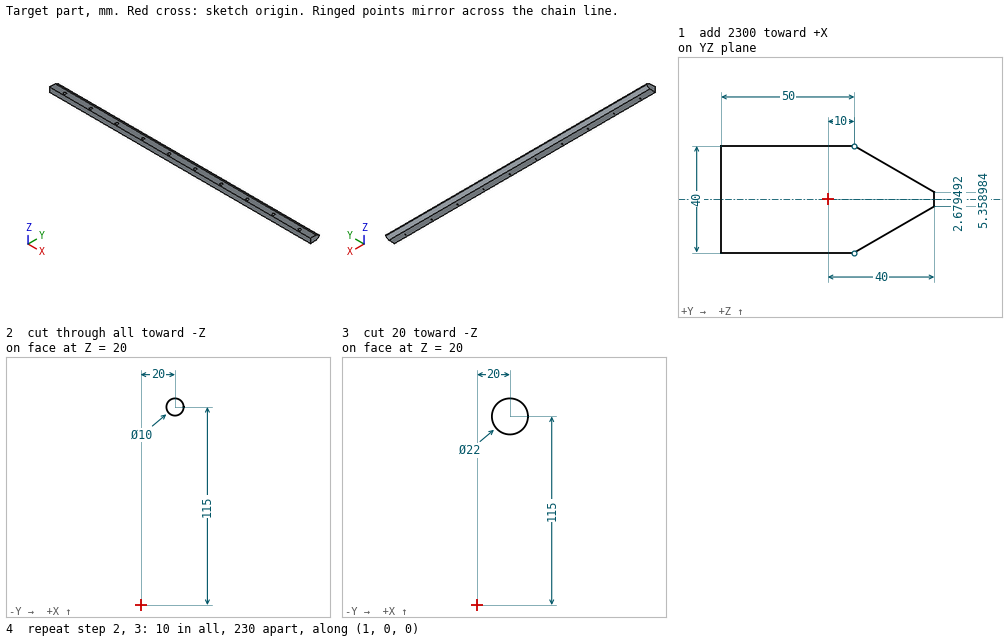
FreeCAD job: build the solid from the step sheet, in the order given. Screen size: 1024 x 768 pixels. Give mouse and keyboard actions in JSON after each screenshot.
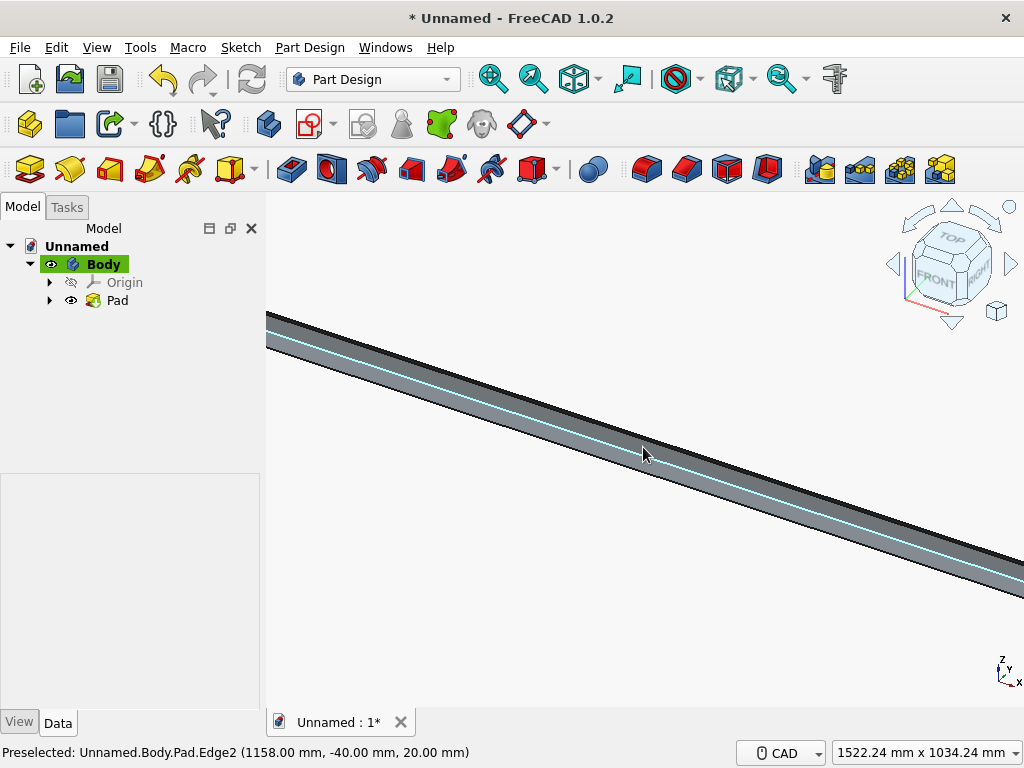
{"action": "key", "text": "v f"}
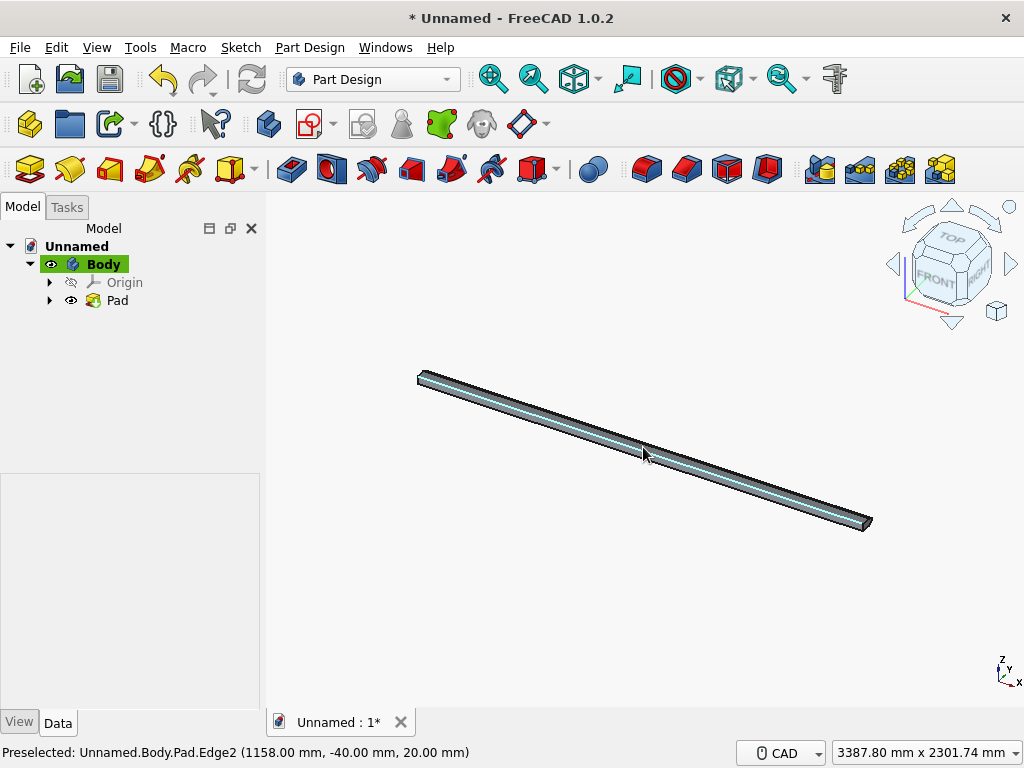
{"action": "key", "text": "0"}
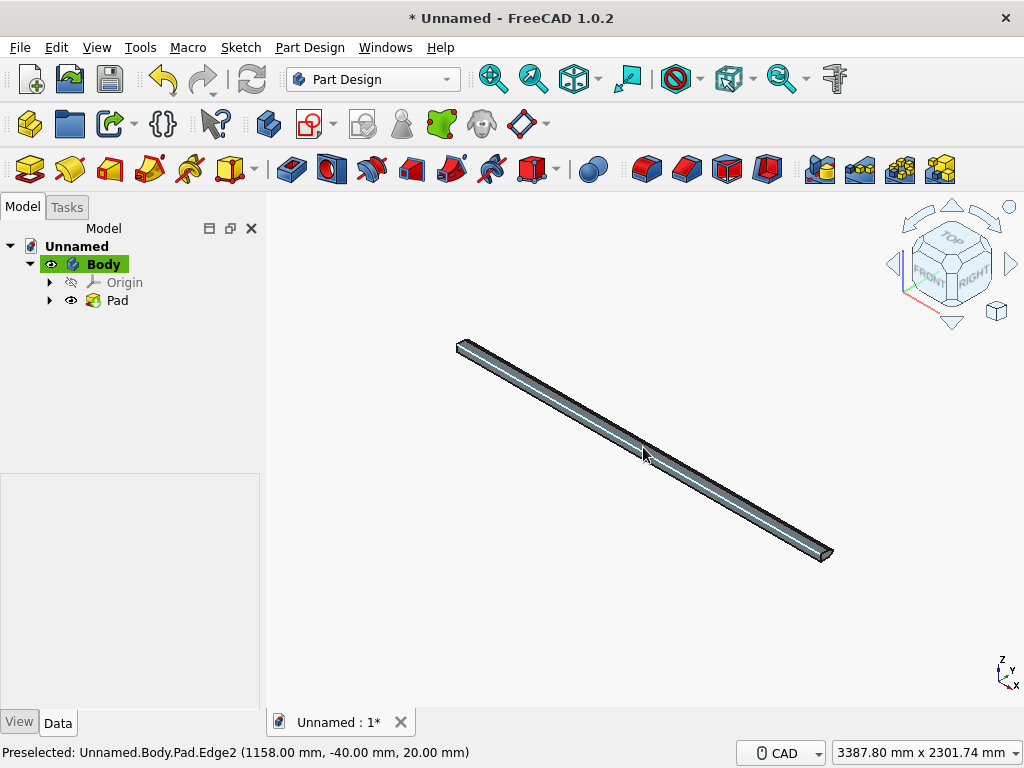
{"action": "scroll", "coordinate": [643, 446], "scroll_direction": "up", "scroll_amount": 4}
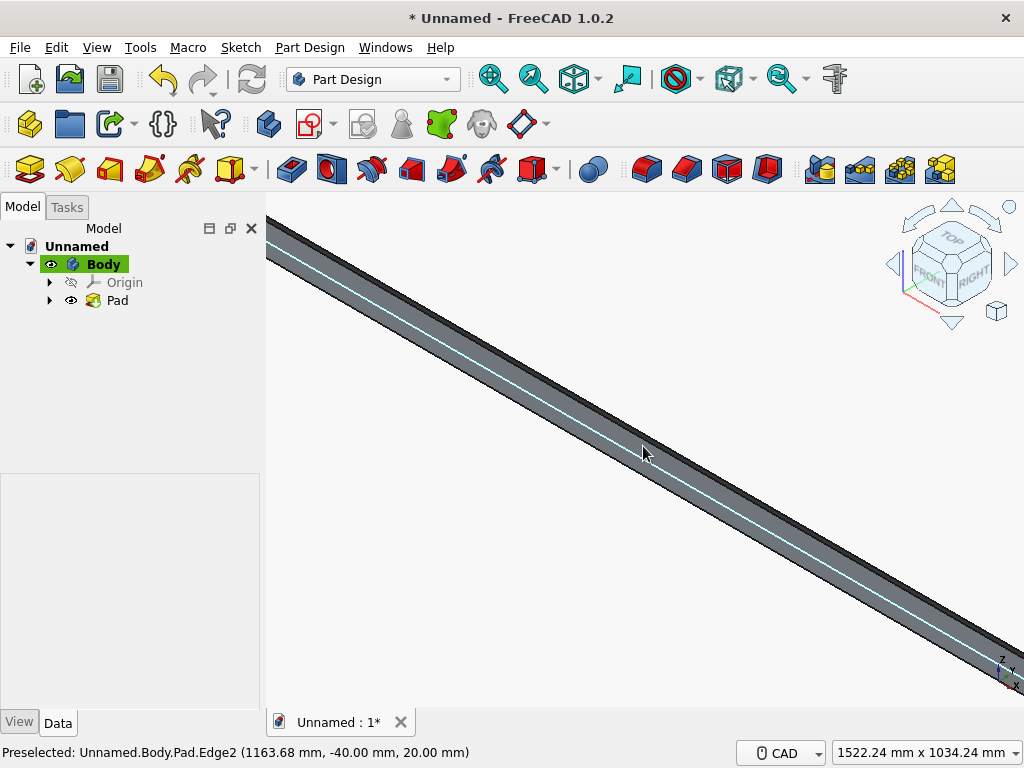
{"action": "left_click", "coordinate": [642, 447]}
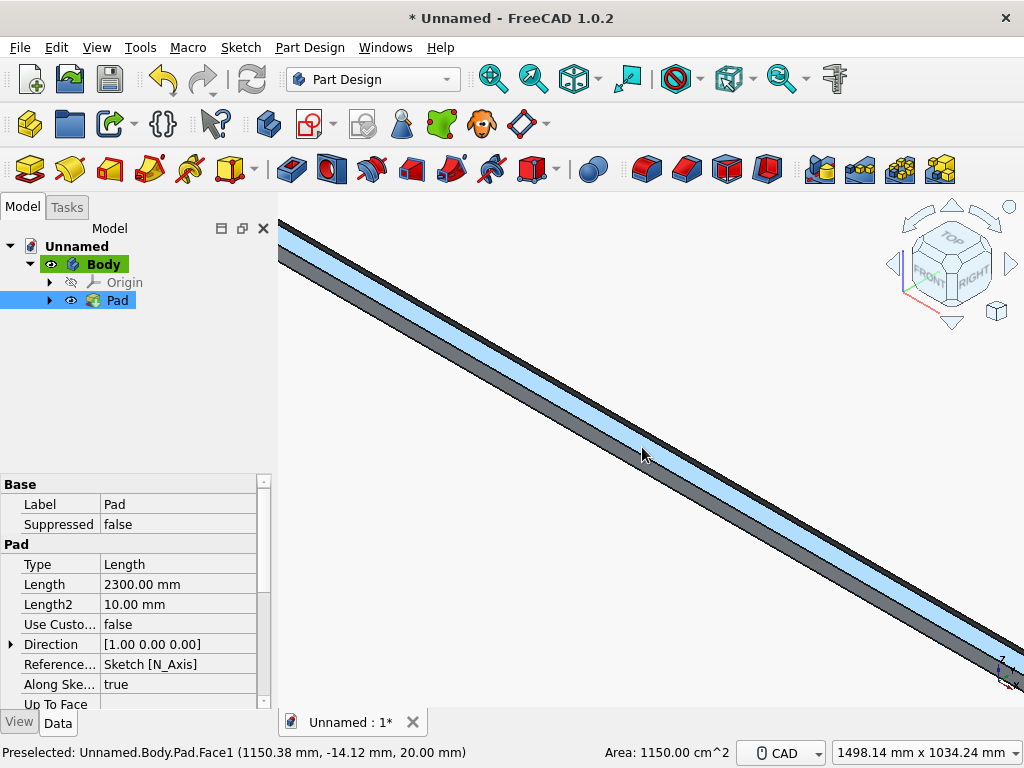
{"action": "left_click", "coordinate": [310, 124]}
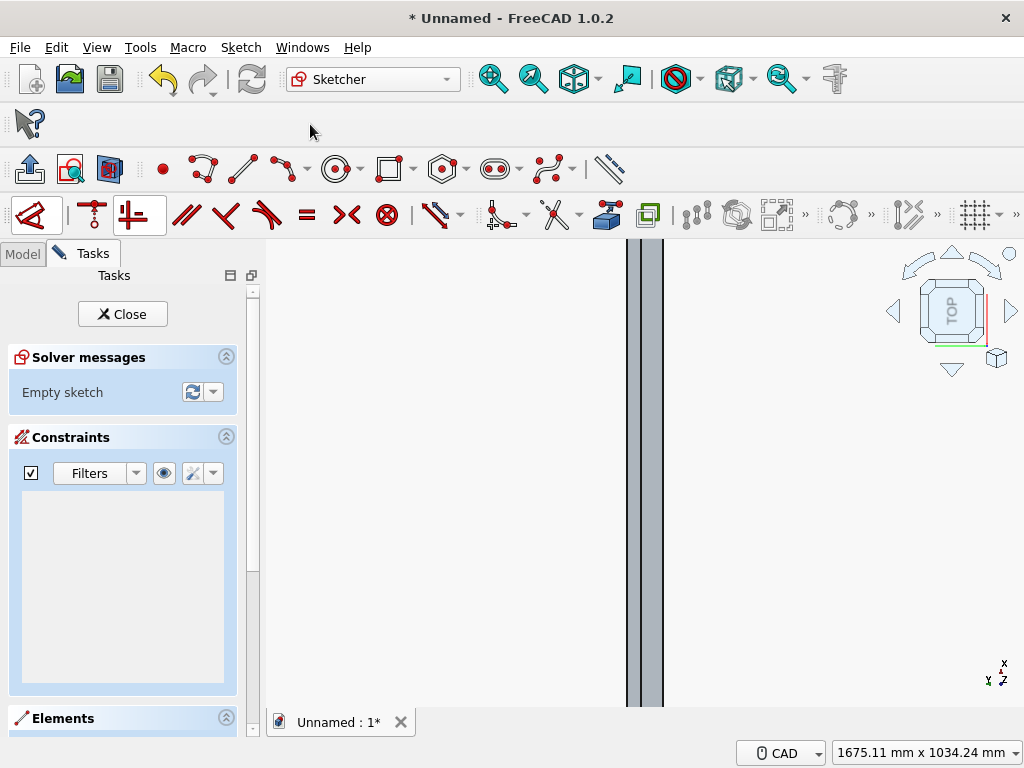
{"action": "scroll", "coordinate": [576, 473], "scroll_direction": "down", "scroll_amount": 5}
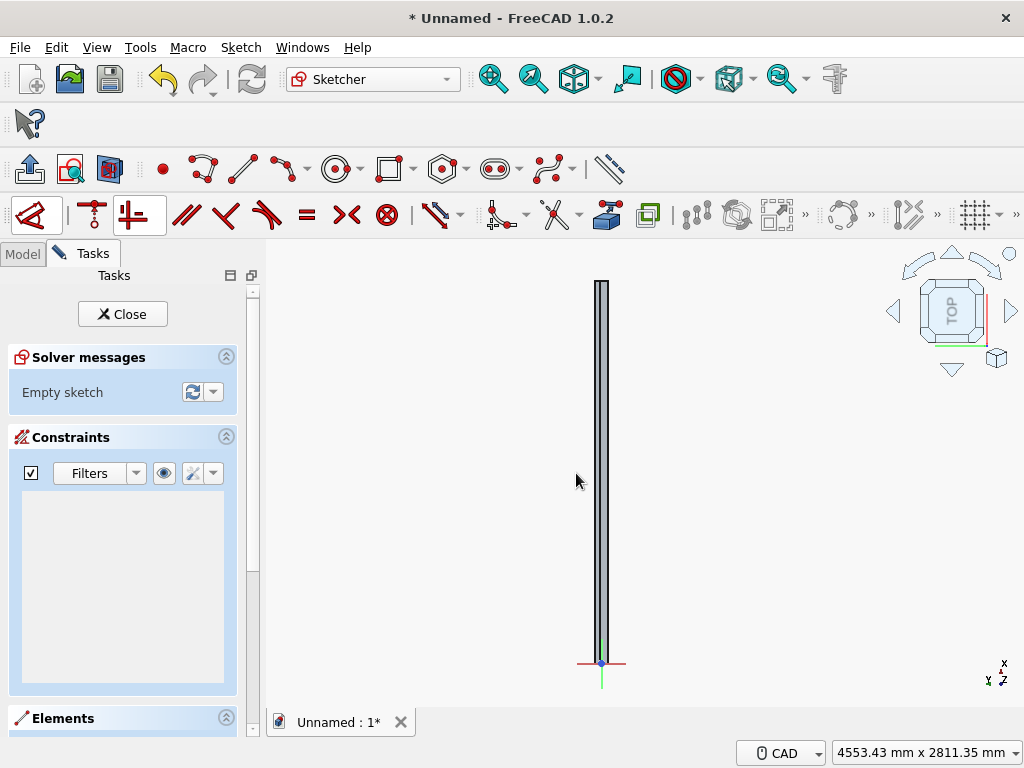
{"action": "scroll", "coordinate": [607, 654], "scroll_direction": "up", "scroll_amount": 15}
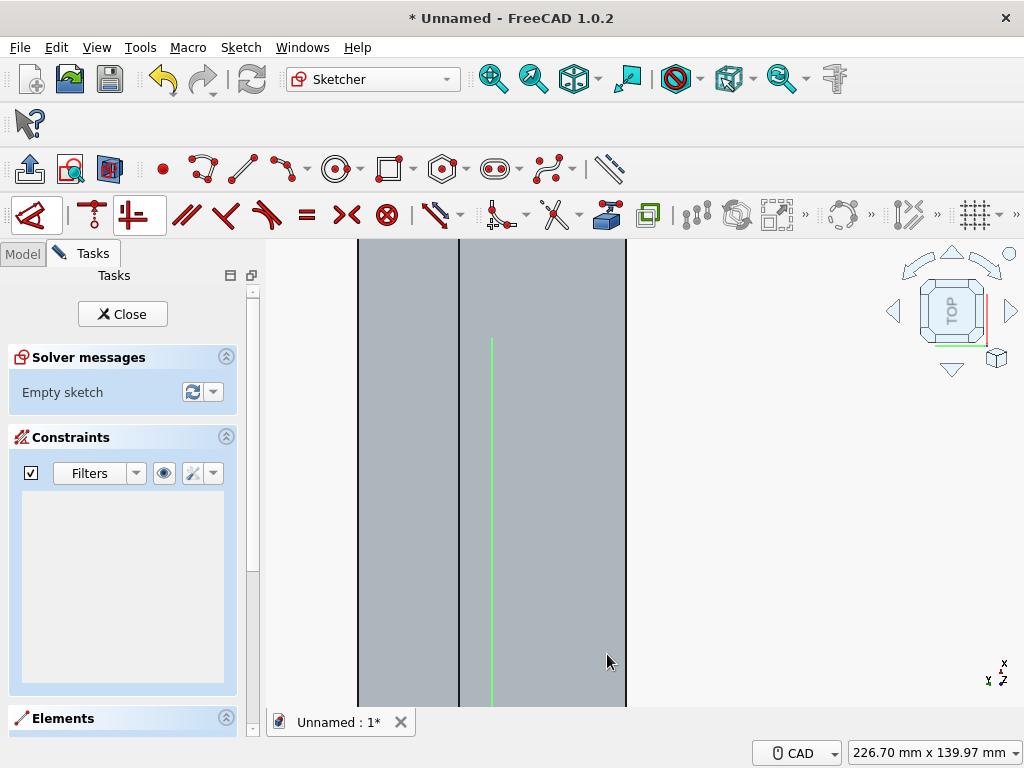
{"action": "scroll", "coordinate": [557, 447], "scroll_direction": "up", "scroll_amount": 11}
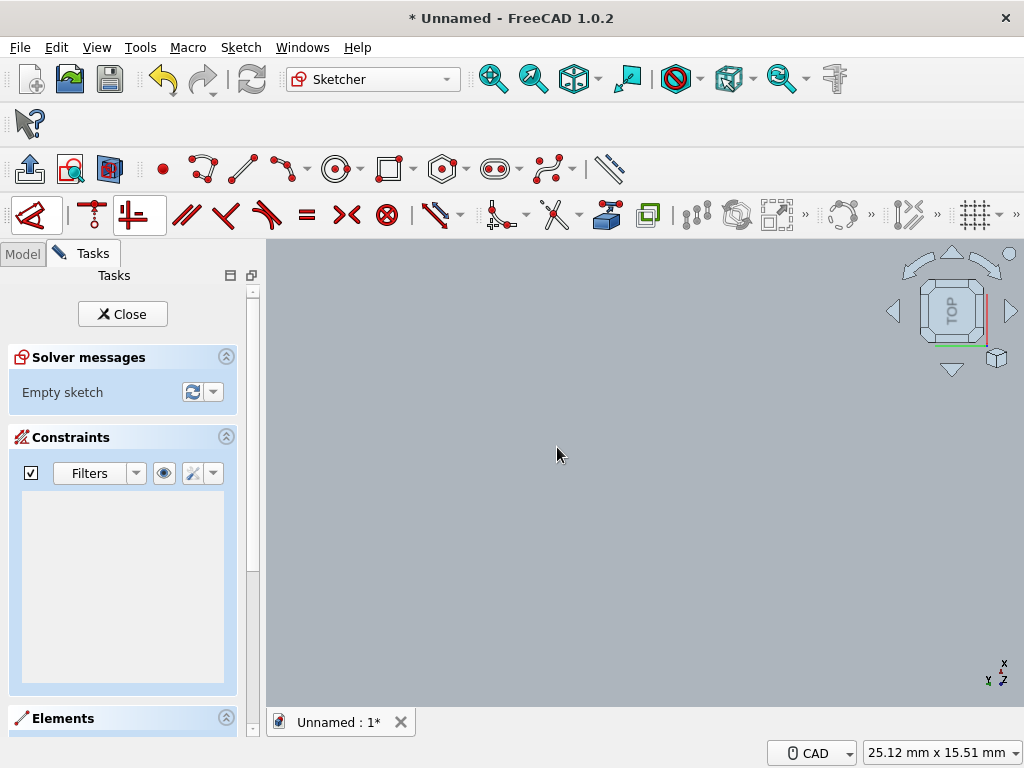
{"action": "key", "text": "g c"}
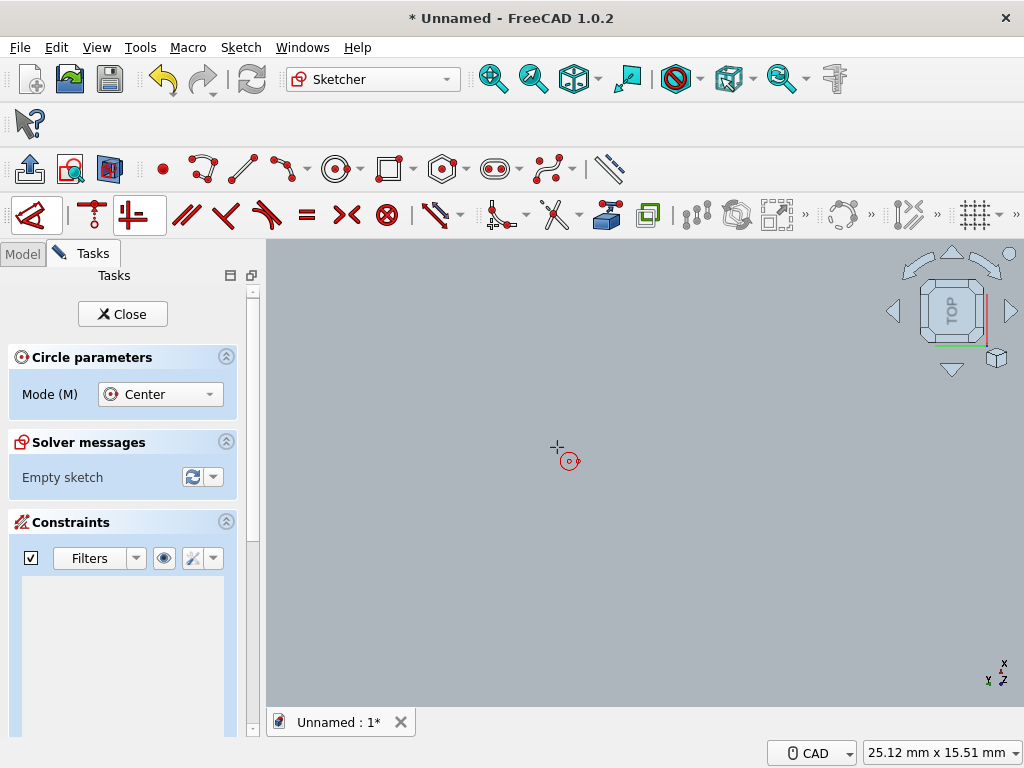
{"action": "left_click", "coordinate": [572, 468]}
{"action": "mouse_move", "coordinate": [679, 361]}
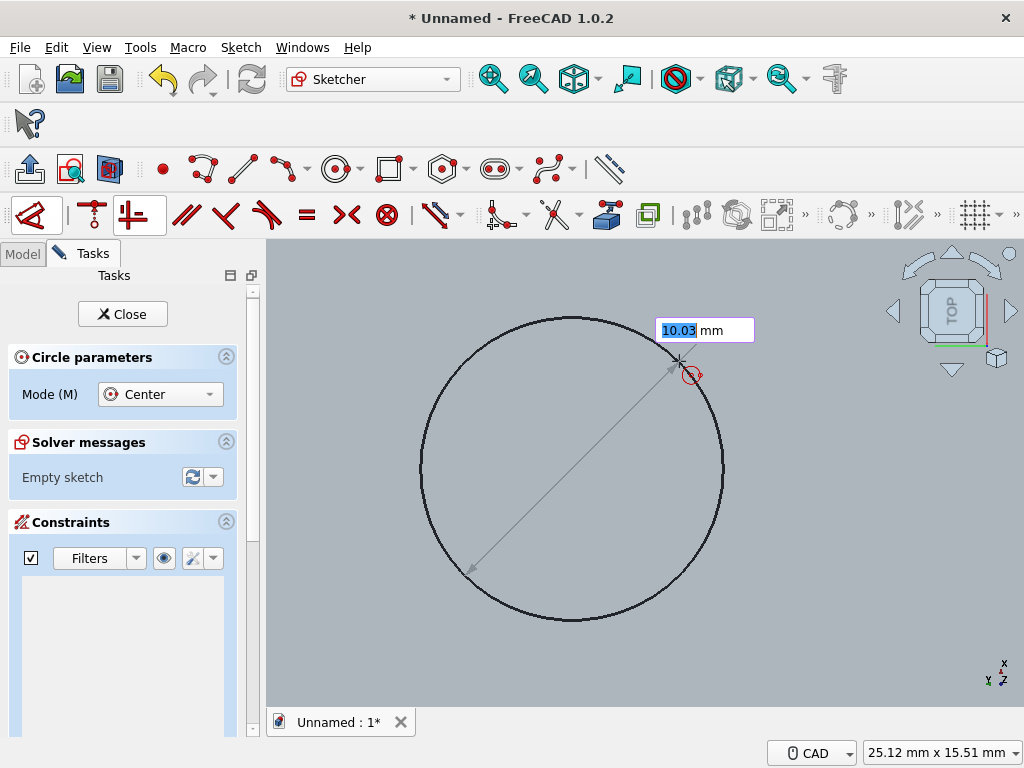
{"action": "type", "text": "10"}
{"action": "key", "text": "Return"}
{"action": "key", "text": "Escape"}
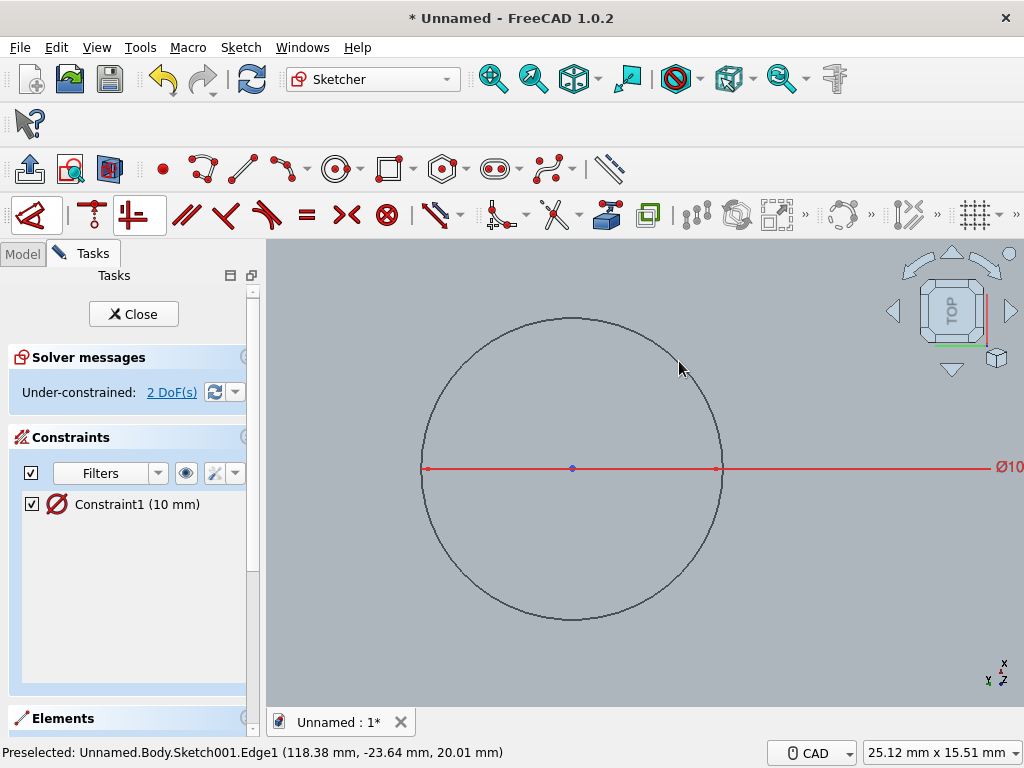
{"action": "left_click", "coordinate": [572, 469]}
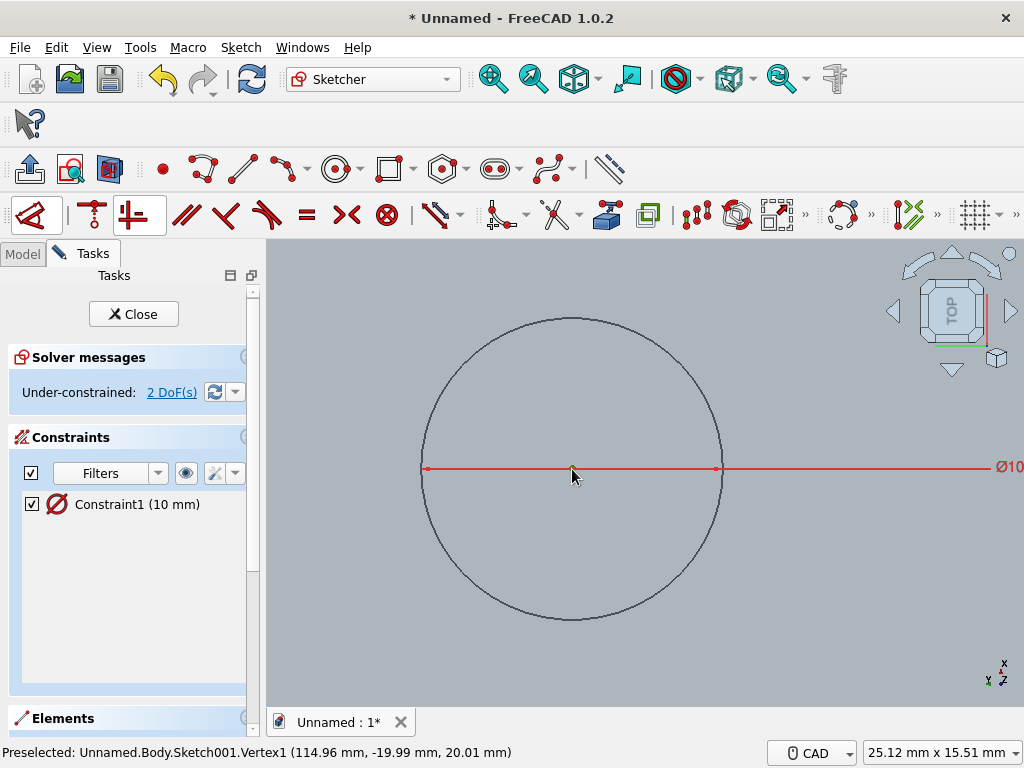
{"action": "key", "text": "l"}